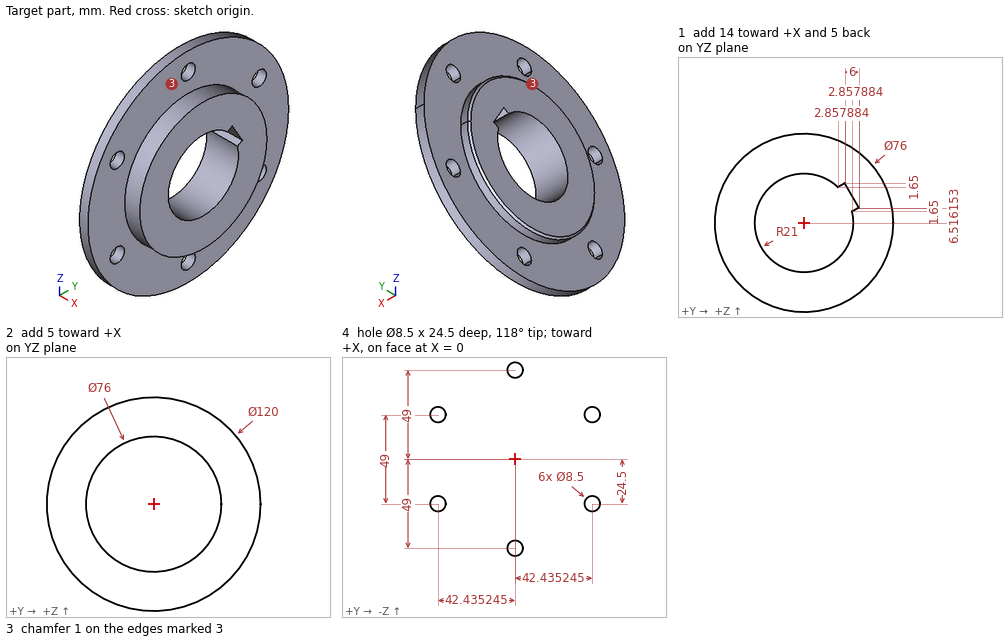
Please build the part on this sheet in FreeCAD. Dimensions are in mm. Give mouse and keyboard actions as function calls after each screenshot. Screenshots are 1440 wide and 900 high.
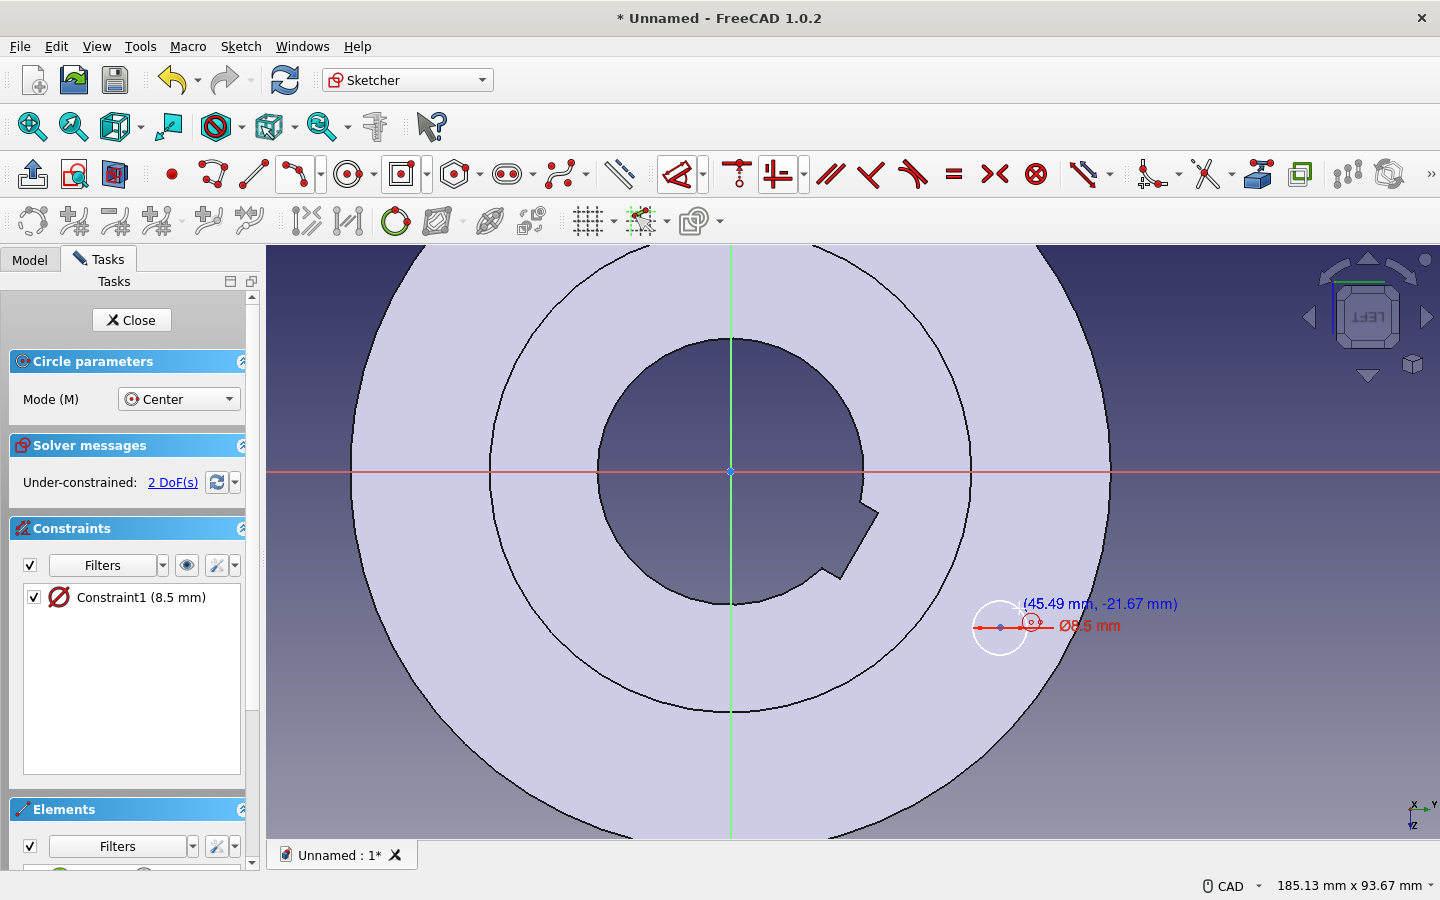
click(731, 782)
move(750, 763)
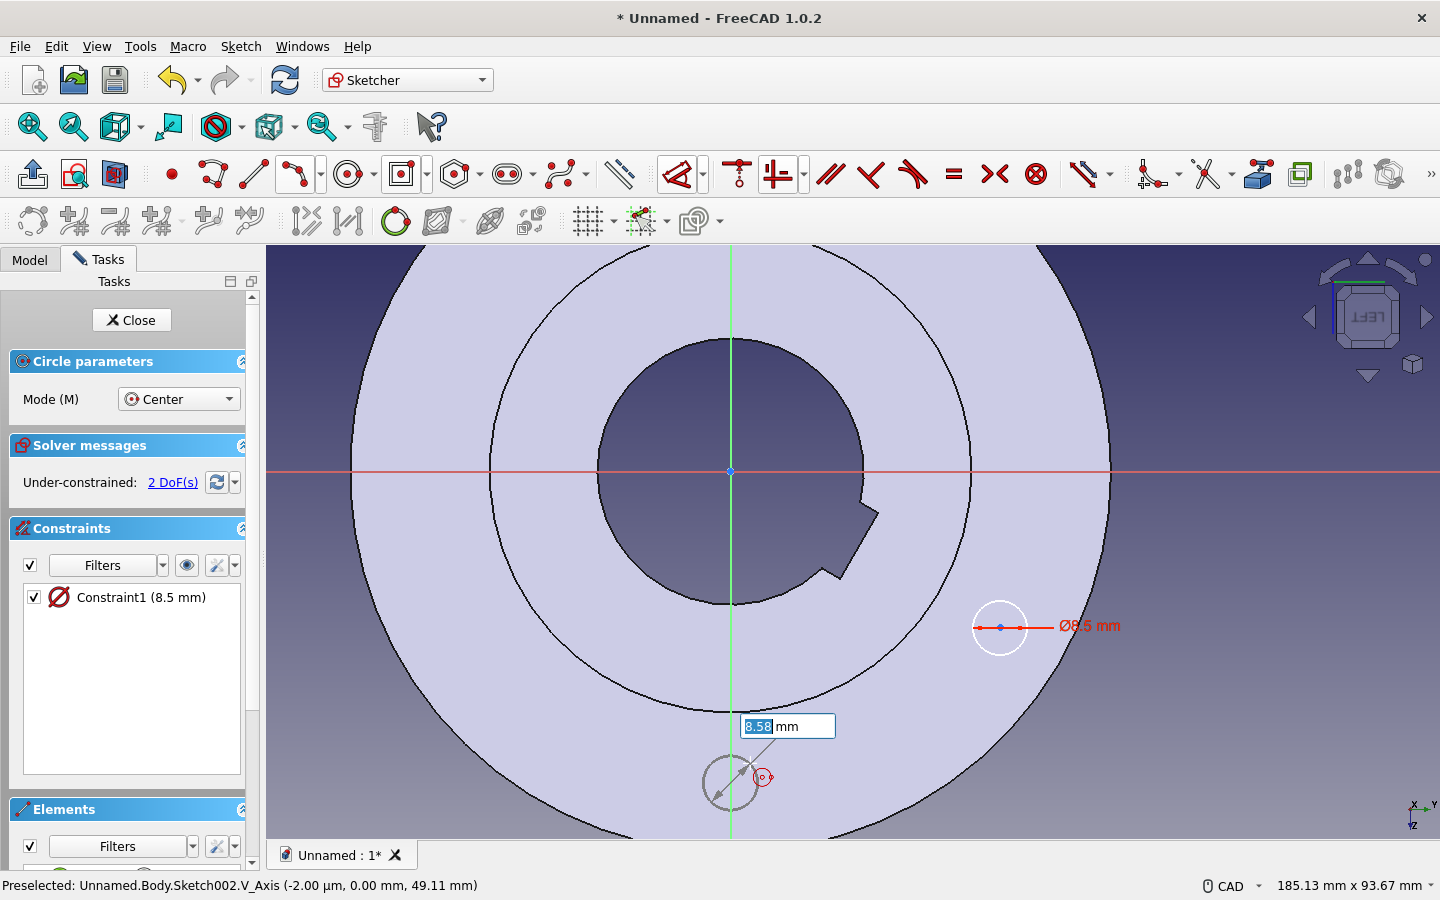
text(8.5)
key(Return)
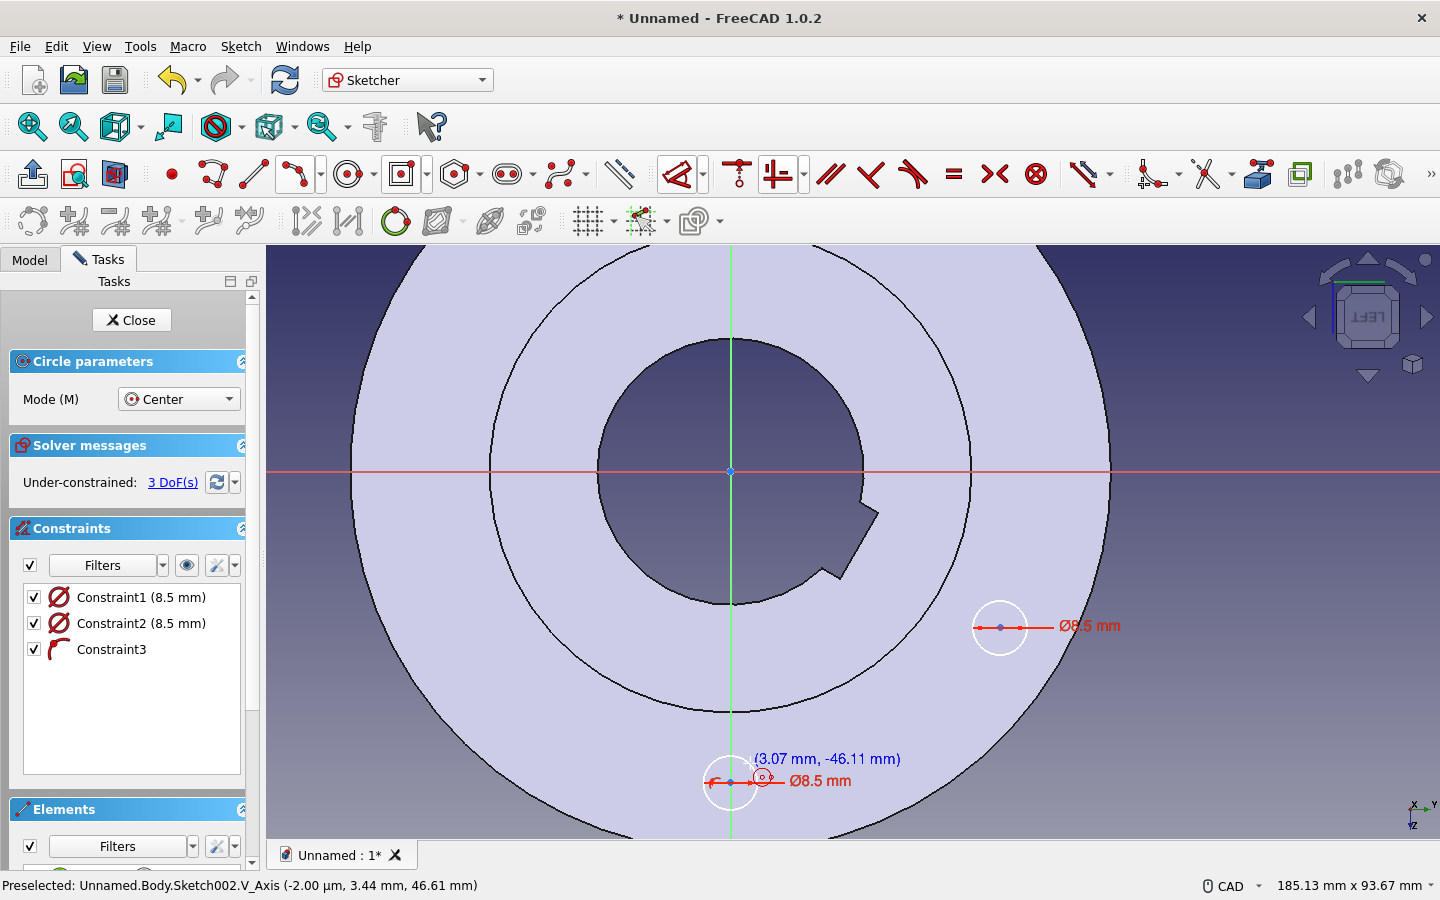
click(461, 627)
move(480, 608)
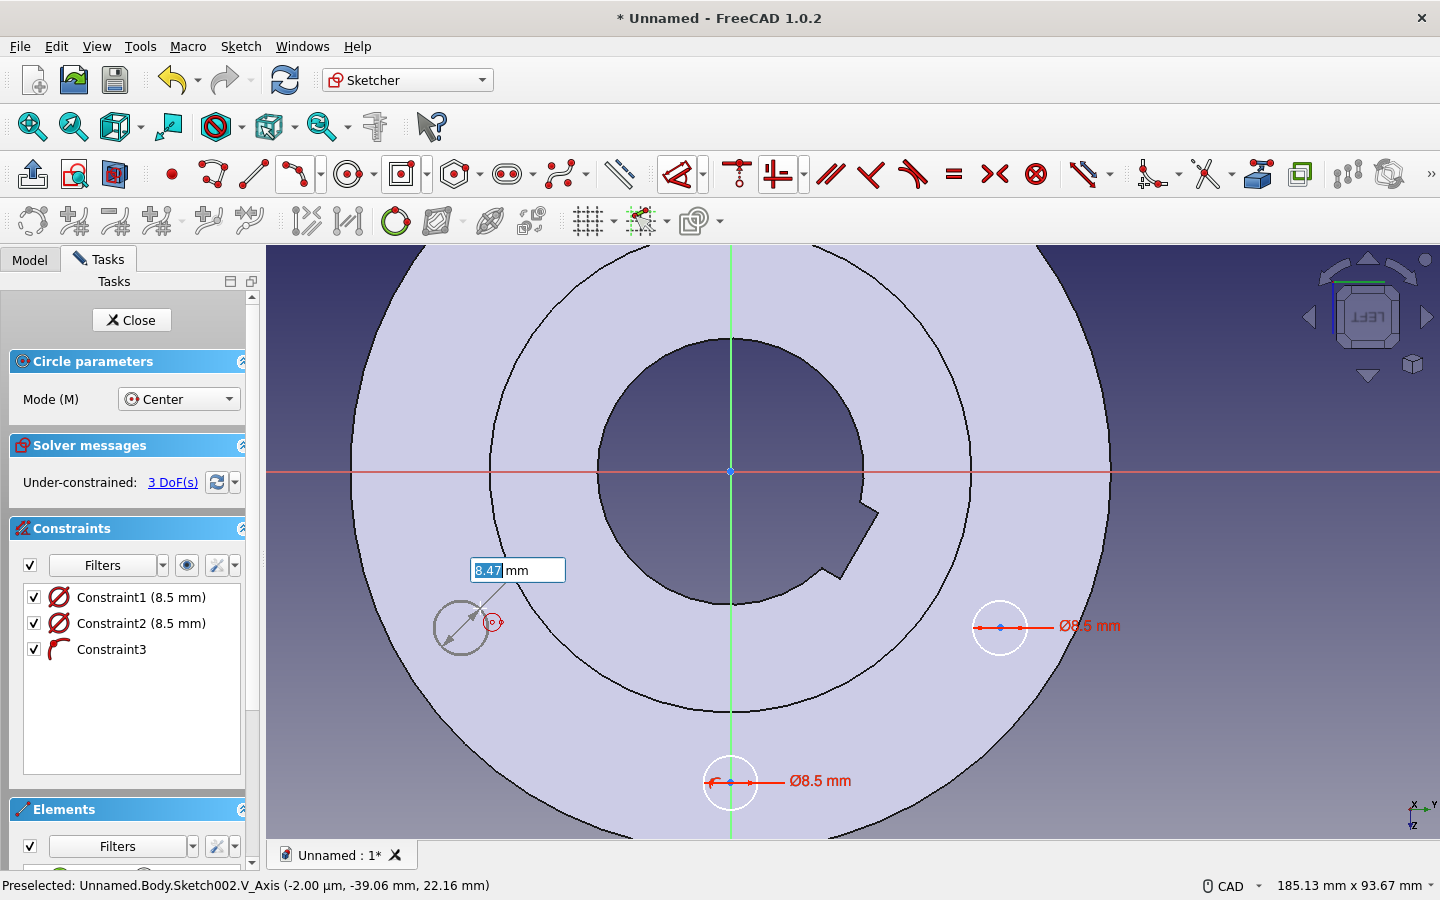
text(8.5)
key(Return)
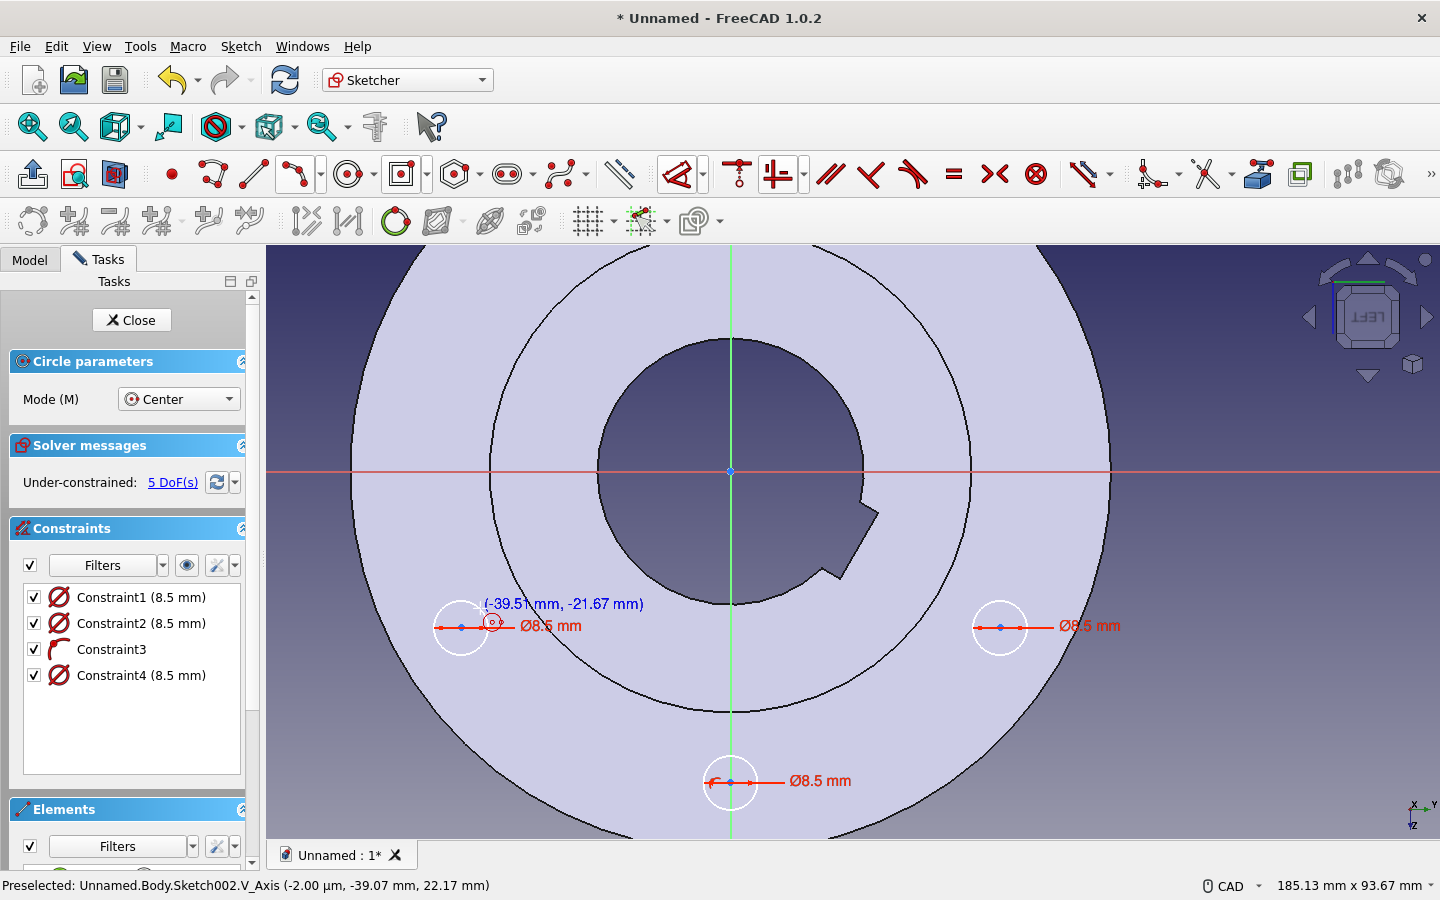
click(461, 316)
move(480, 297)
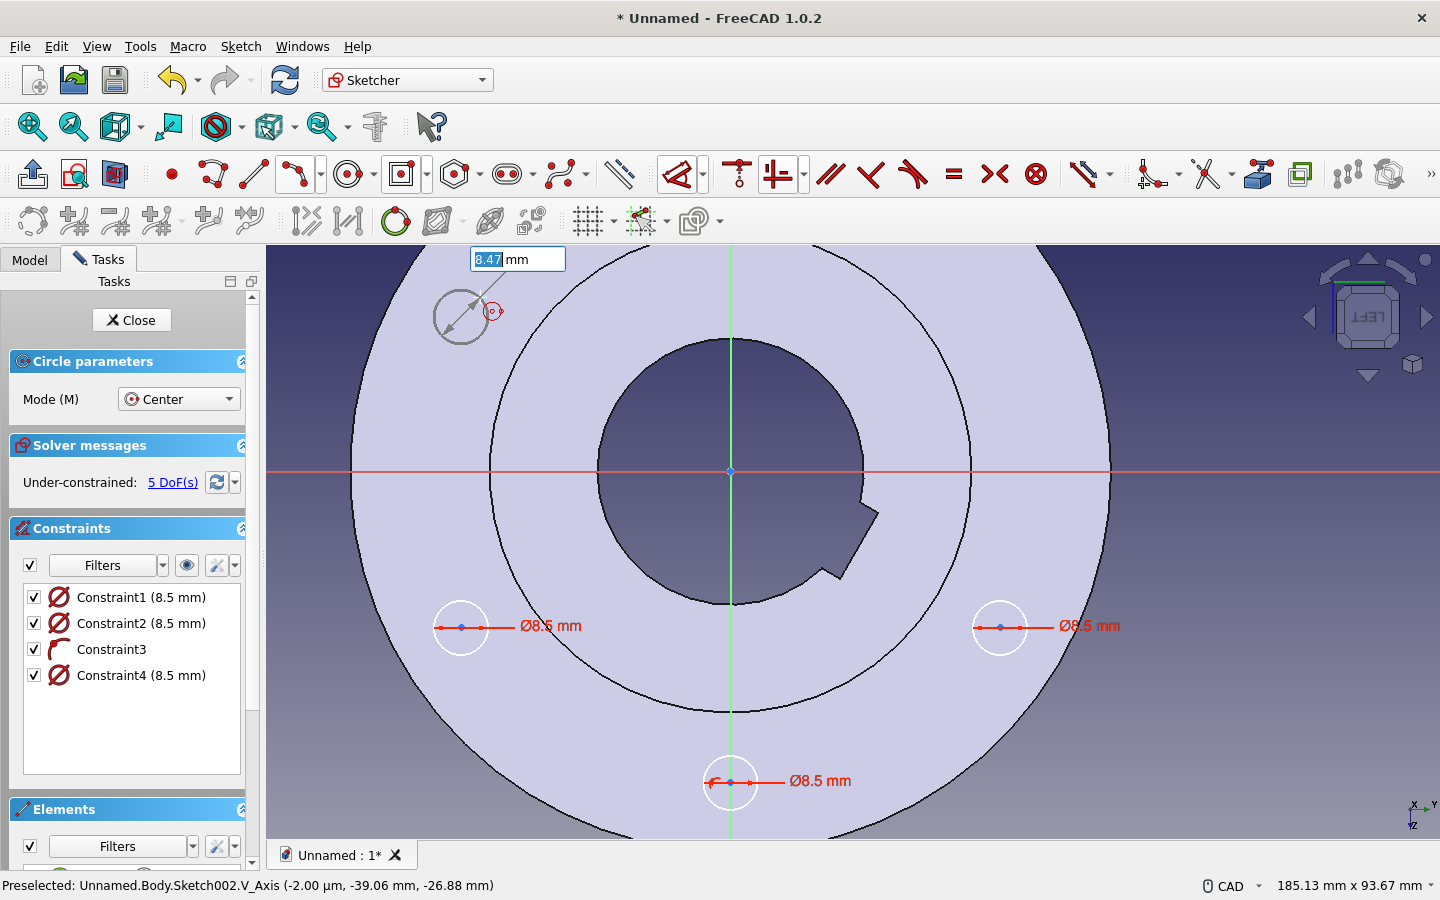
text(8.5)
key(Return)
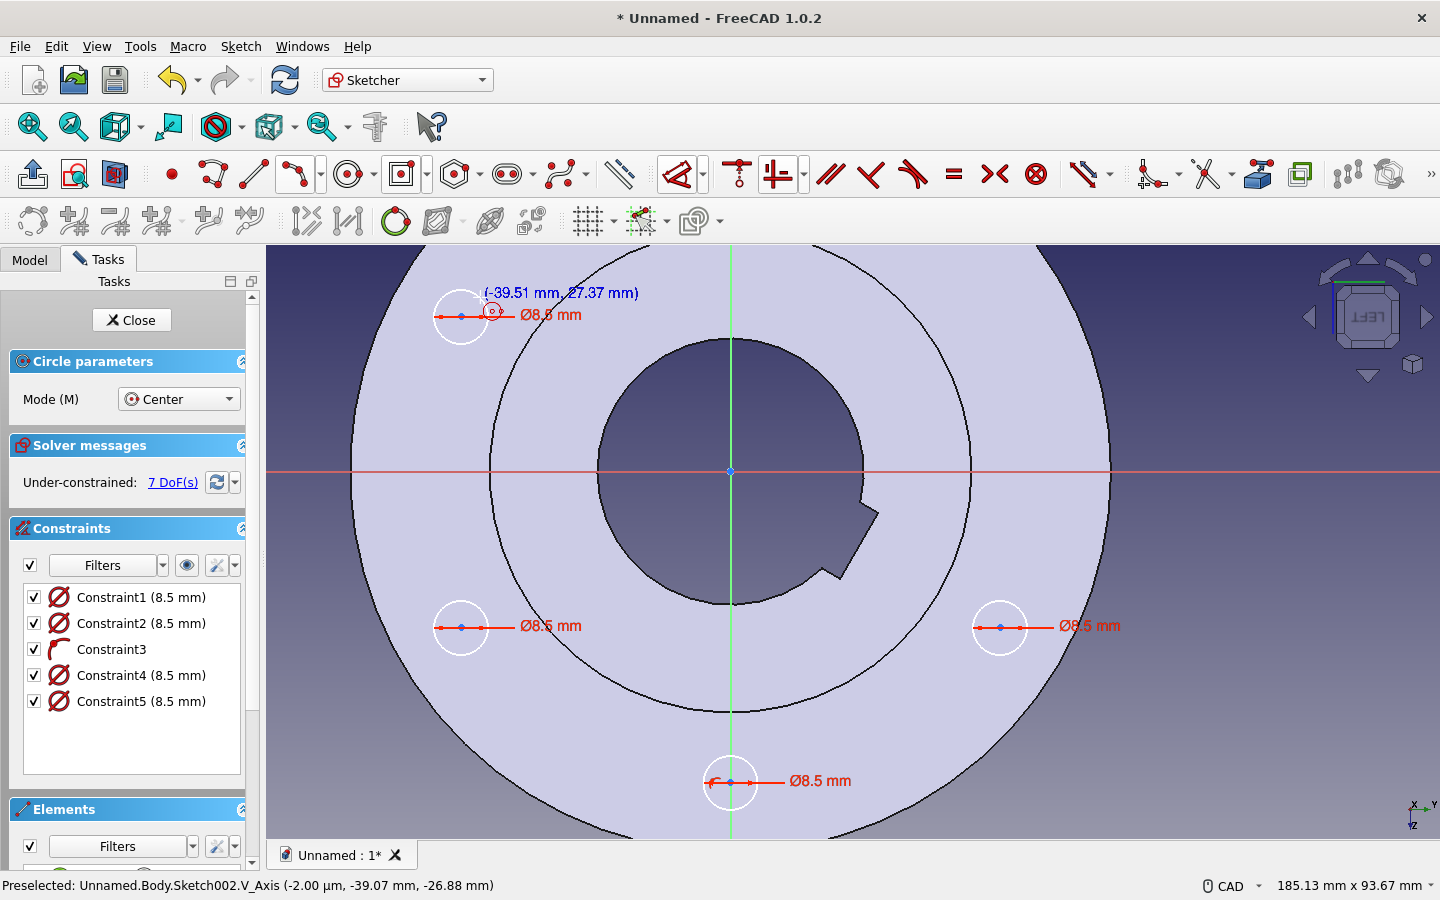
scroll(850, 628, down, 3)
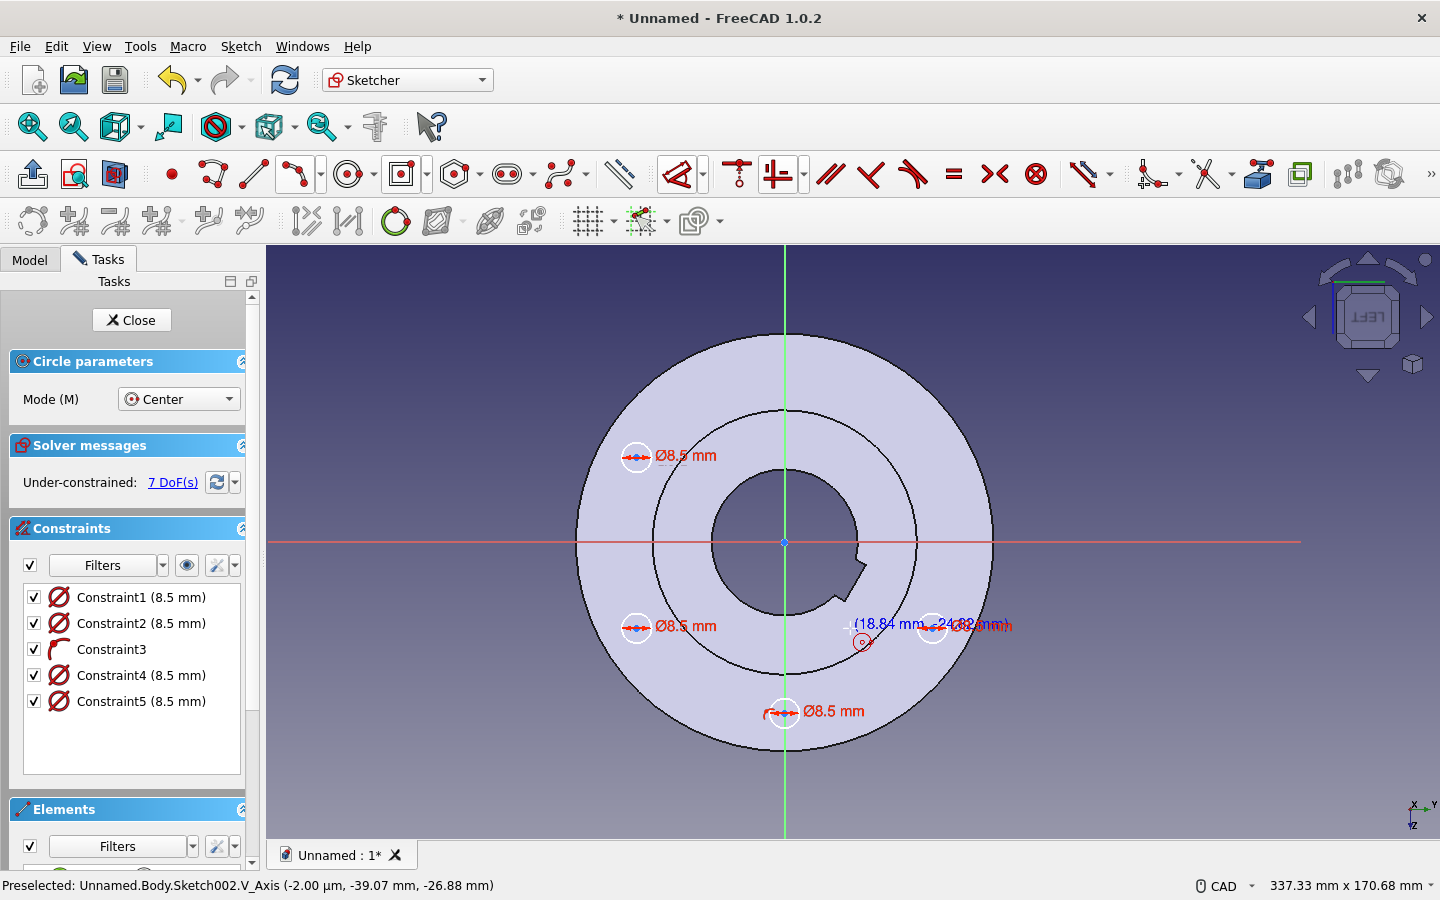
scroll(785, 372, up, 3)